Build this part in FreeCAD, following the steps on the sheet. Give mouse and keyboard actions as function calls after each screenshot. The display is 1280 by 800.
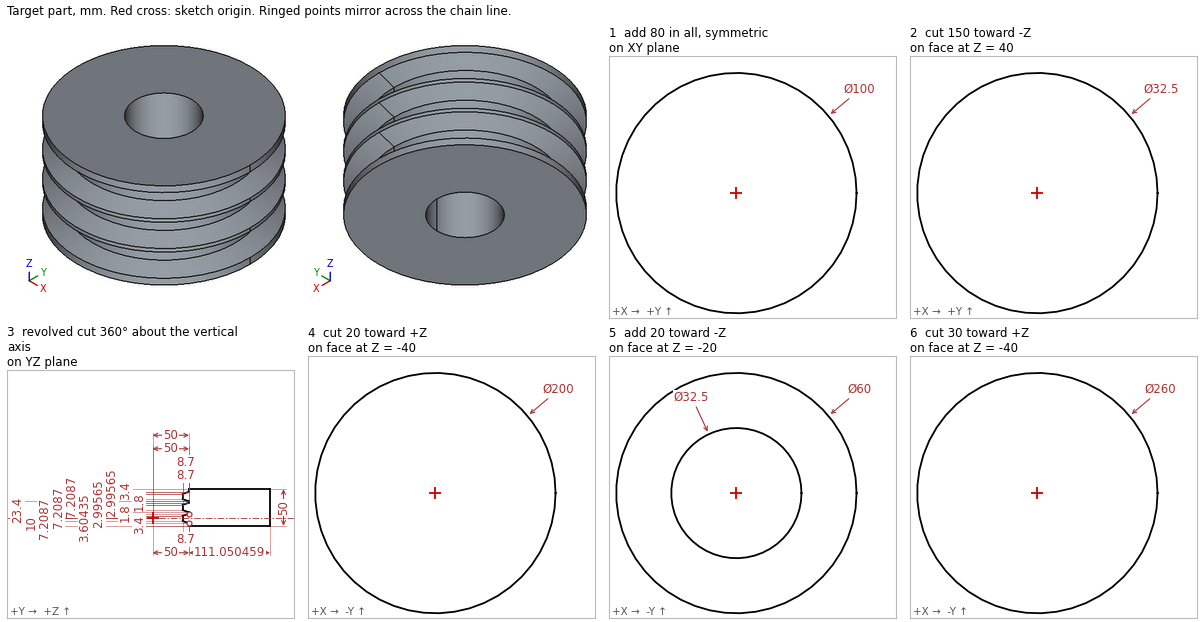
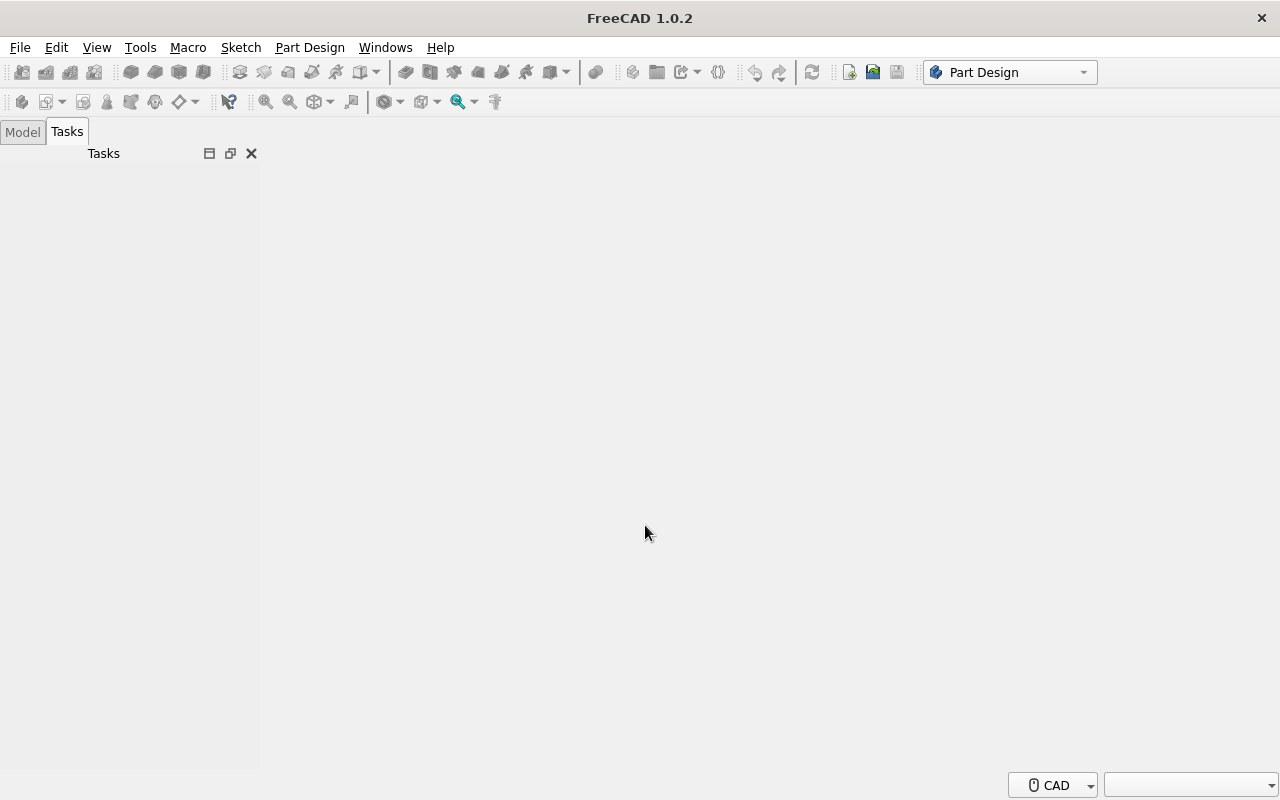
click(850, 72)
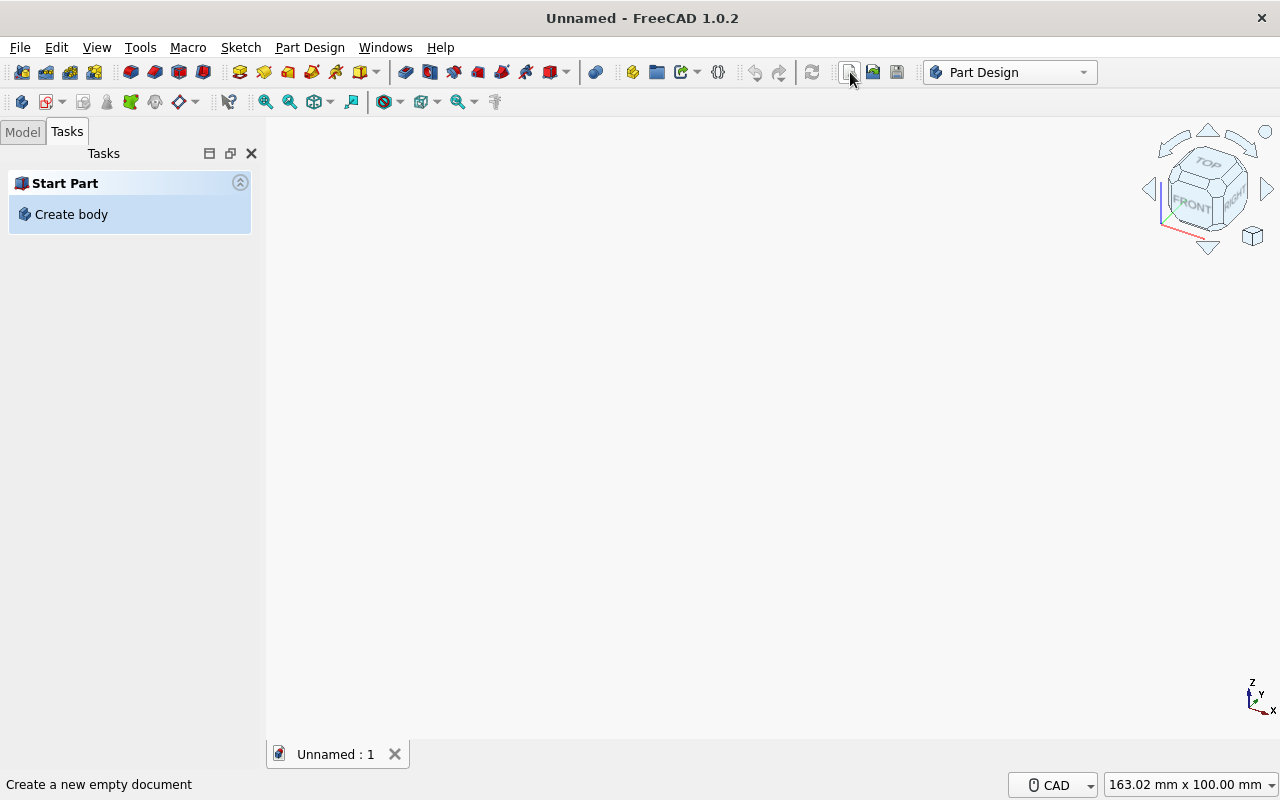
click(46, 102)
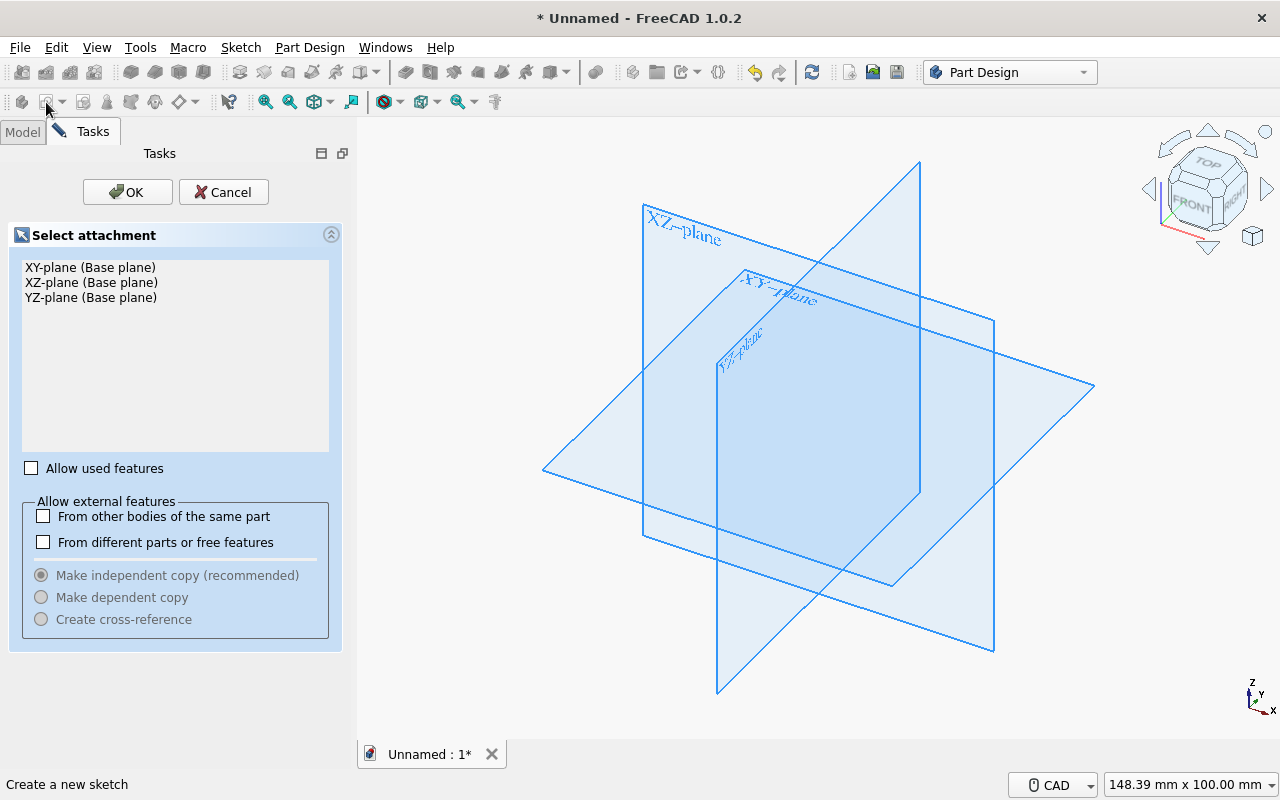
click(82, 268)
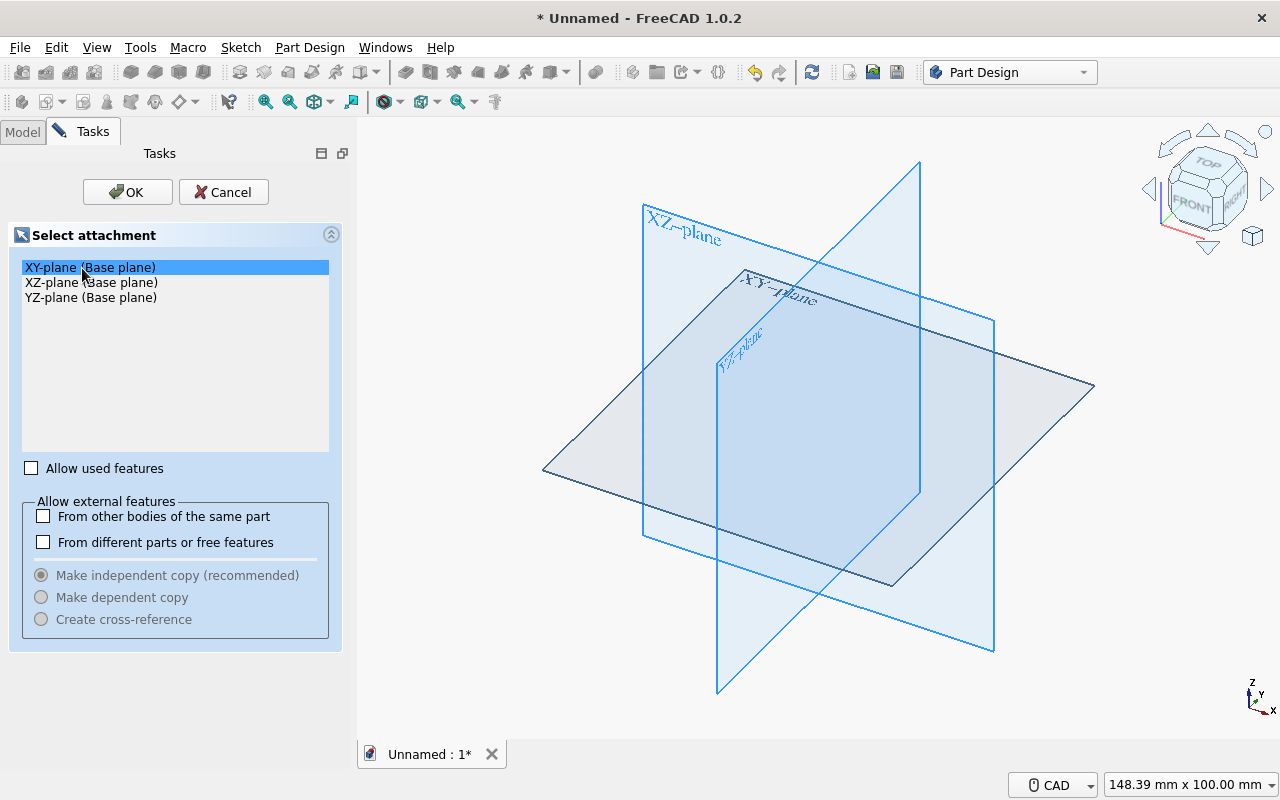
click(128, 192)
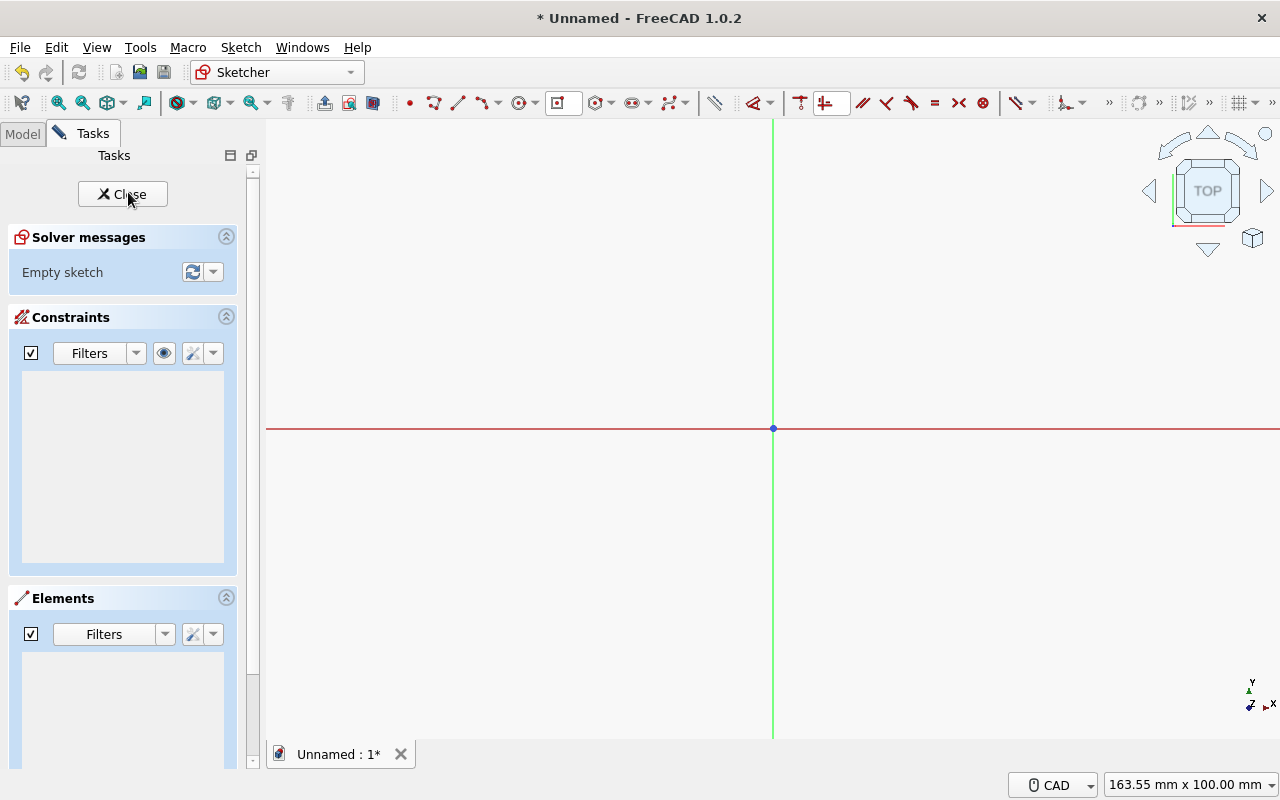
scroll(565, 429, down, 2)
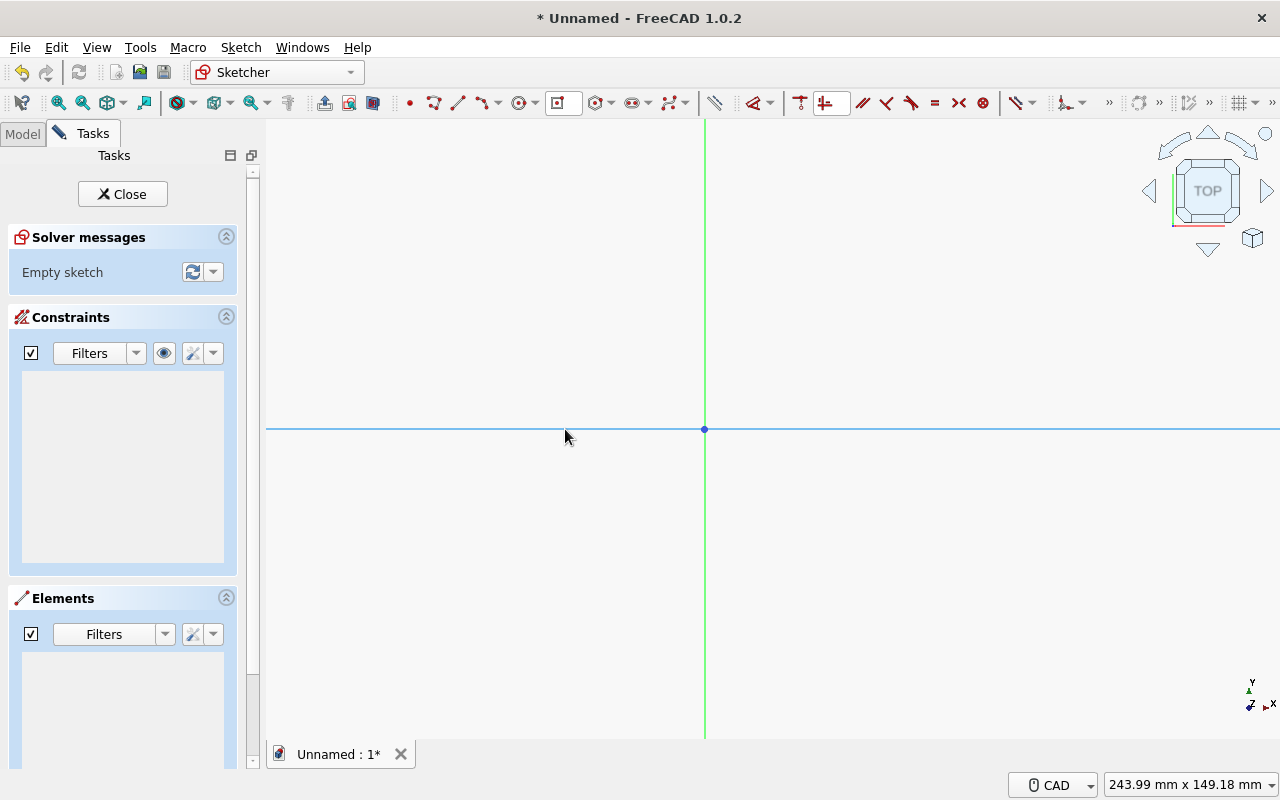
click(520, 104)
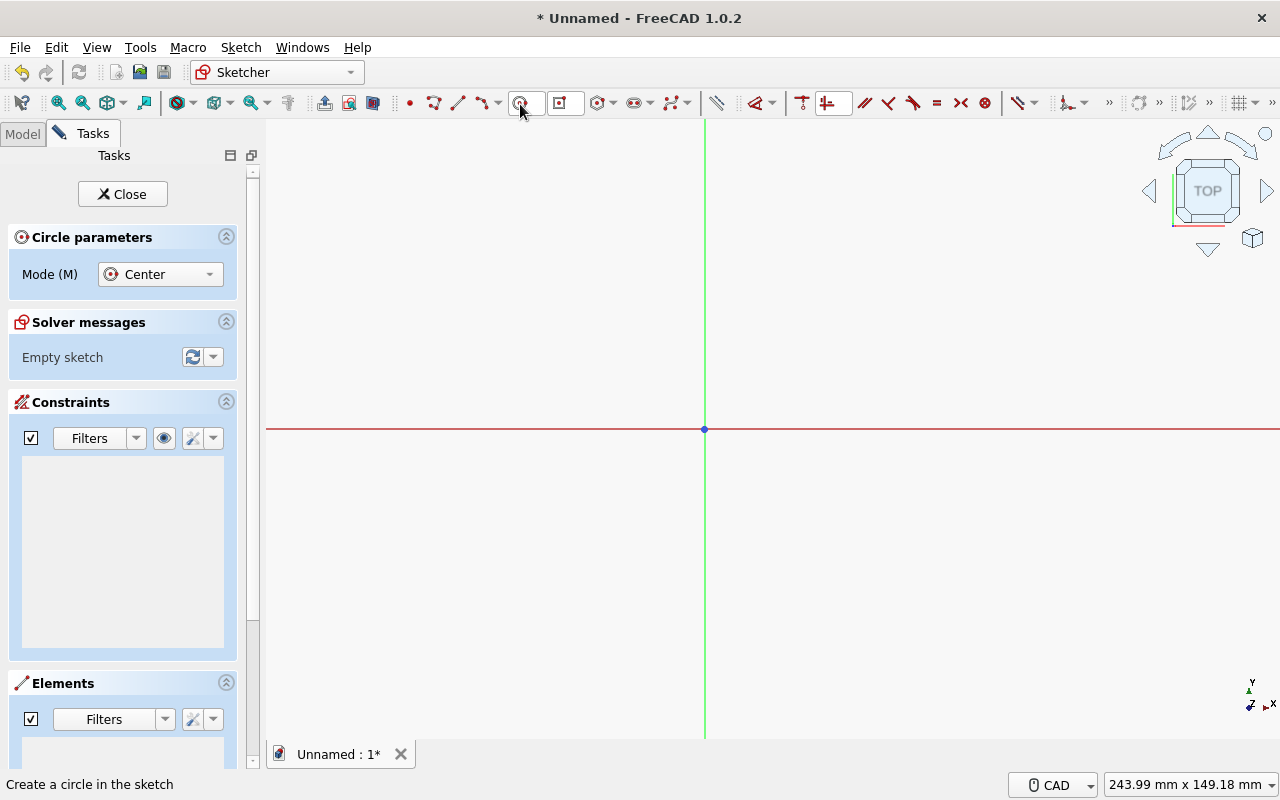
click(705, 429)
click(851, 282)
key(Escape)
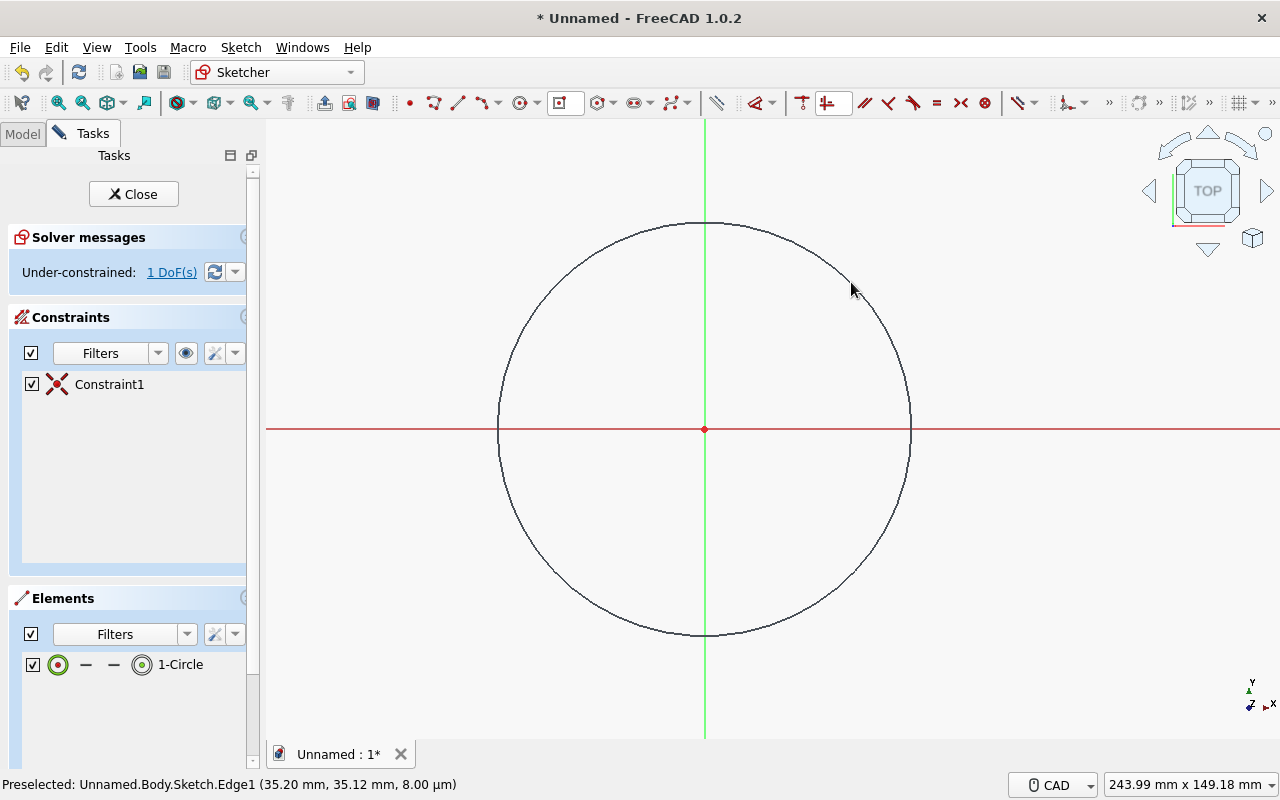
click(756, 104)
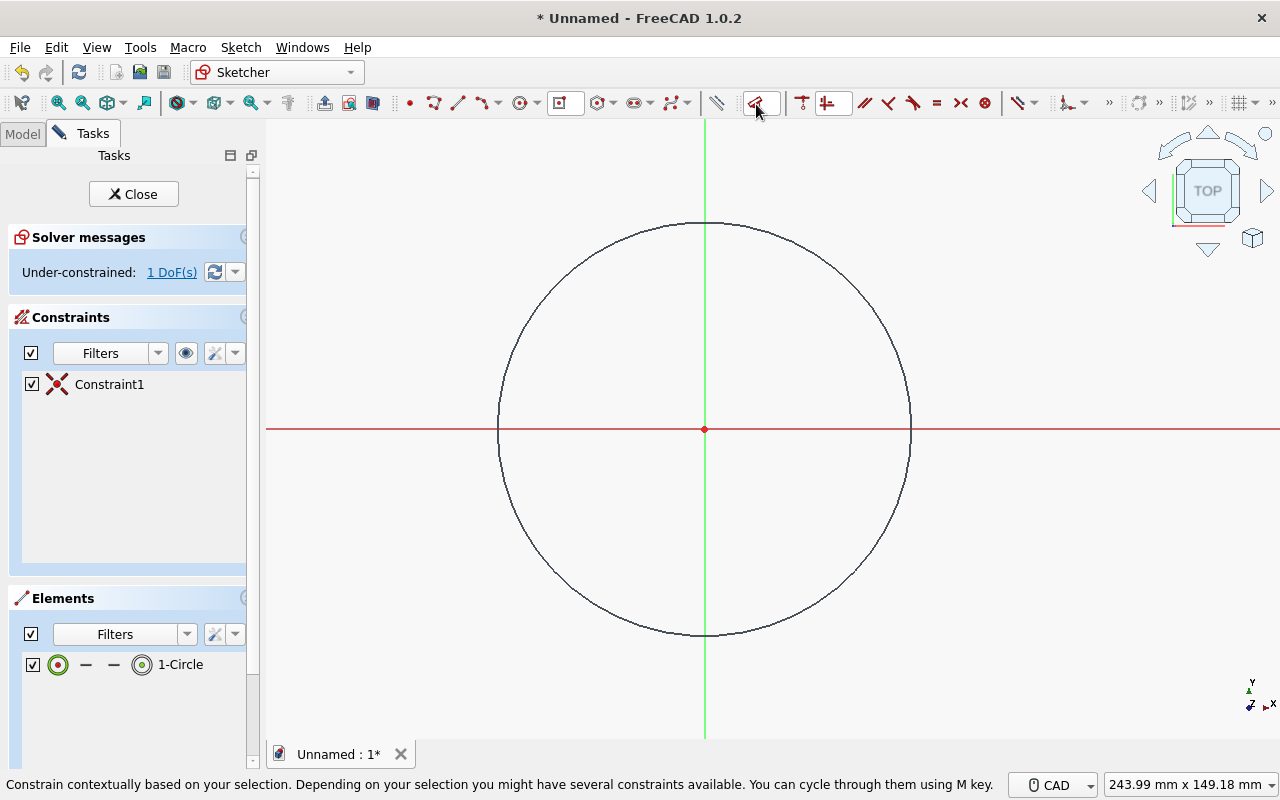
click(850, 282)
click(872, 259)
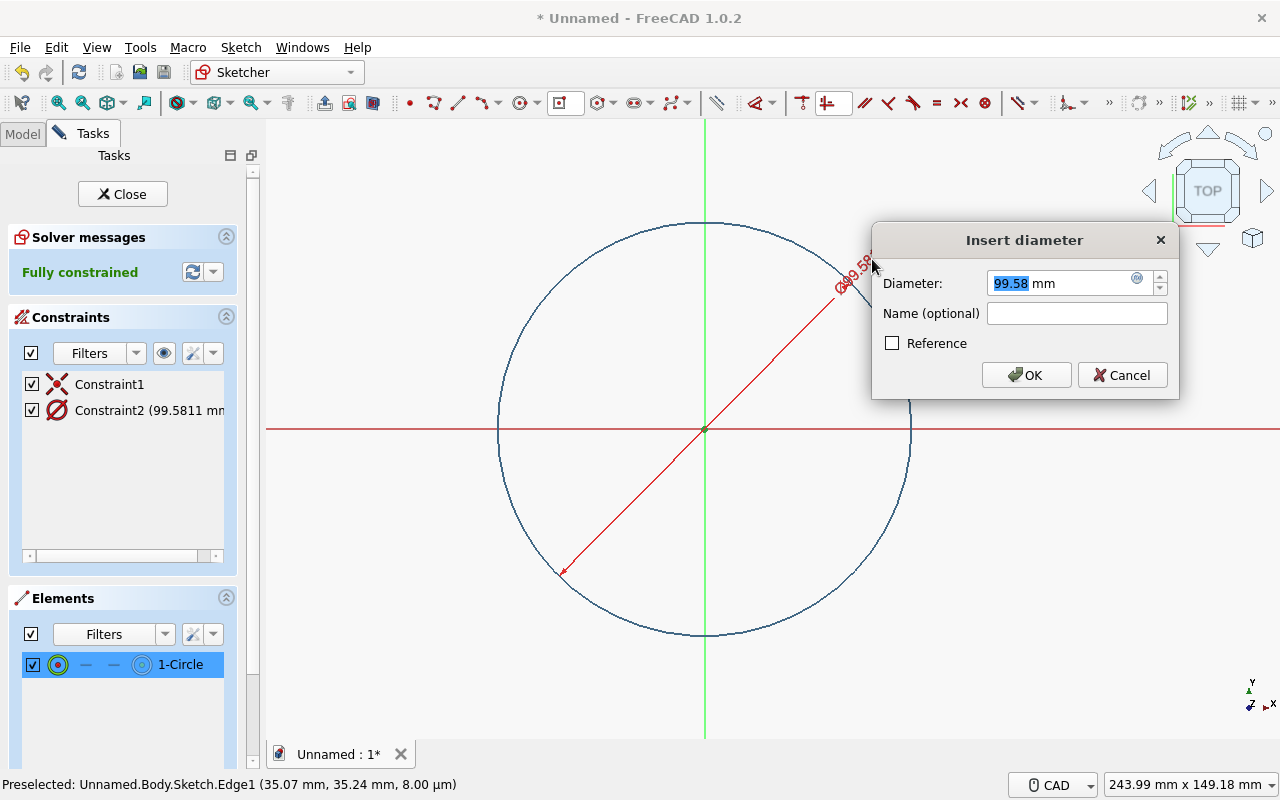
text(100)
key(Return)
key(Escape)